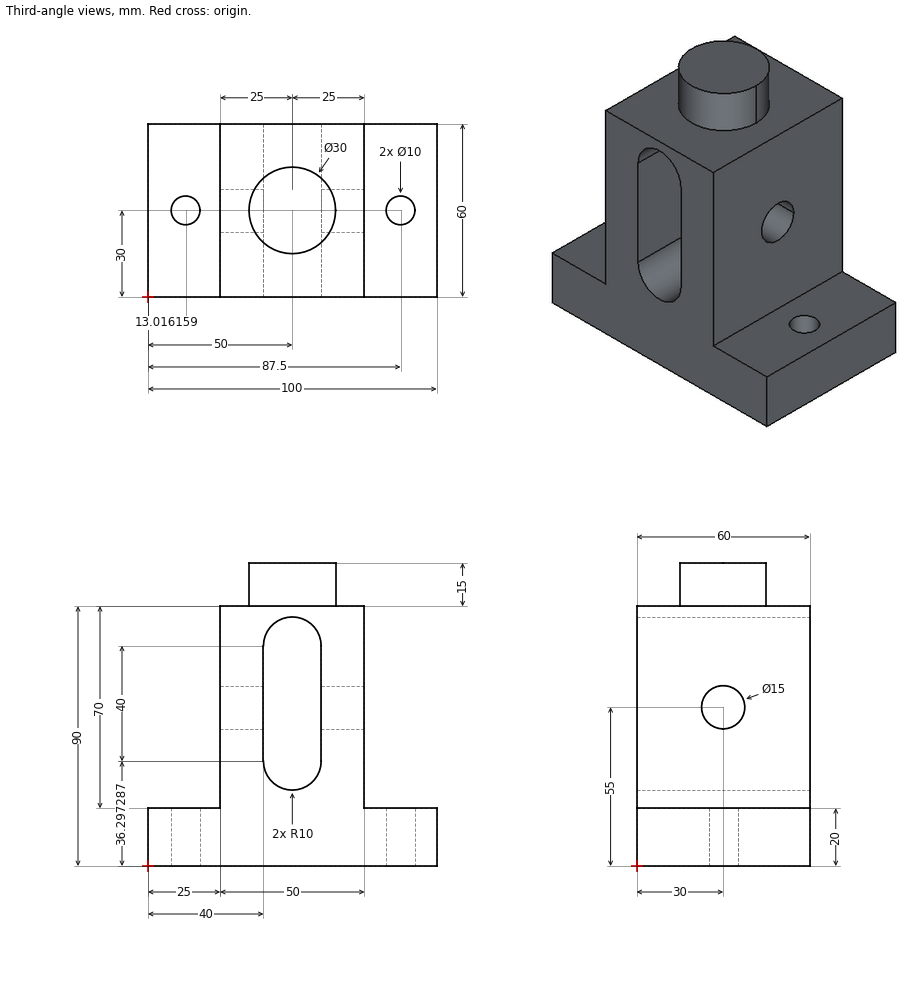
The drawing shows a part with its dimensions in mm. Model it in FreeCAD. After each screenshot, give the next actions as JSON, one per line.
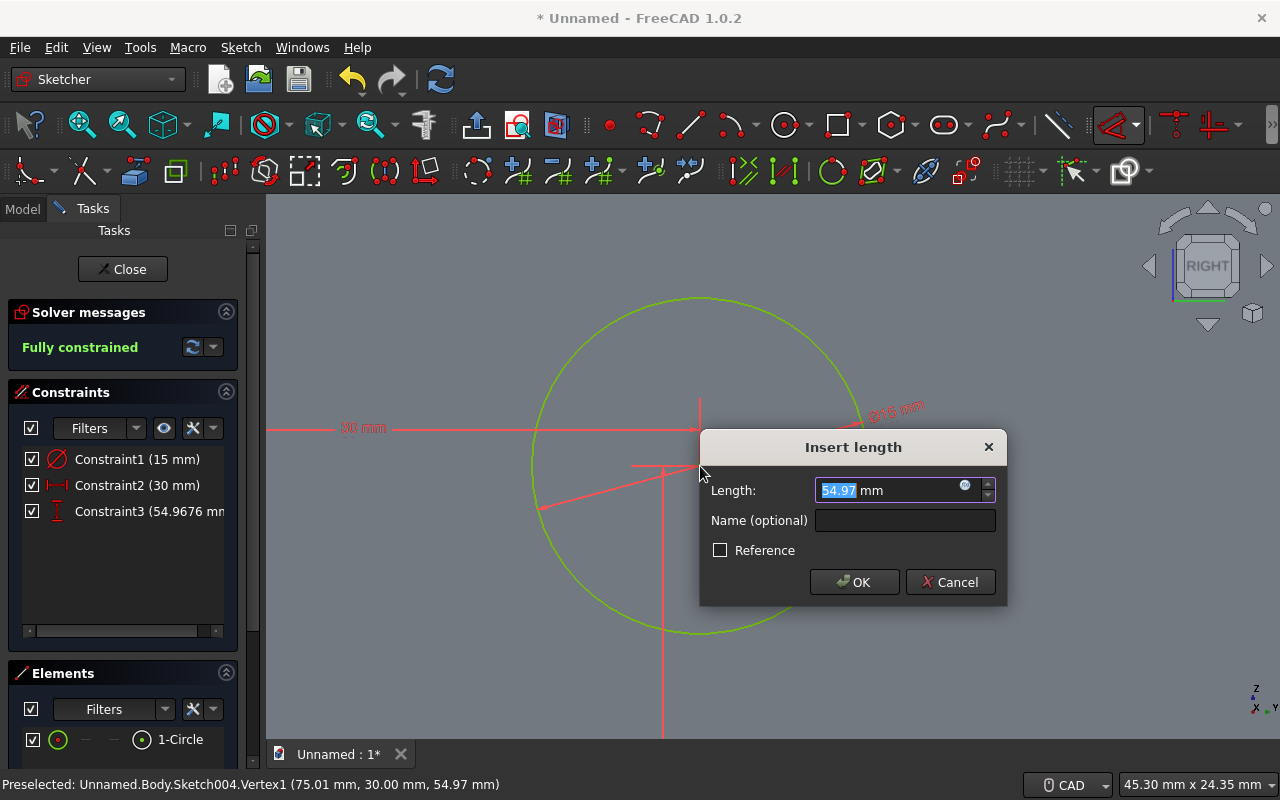
{"action": "type", "text": "55"}
{"action": "key", "text": "Return"}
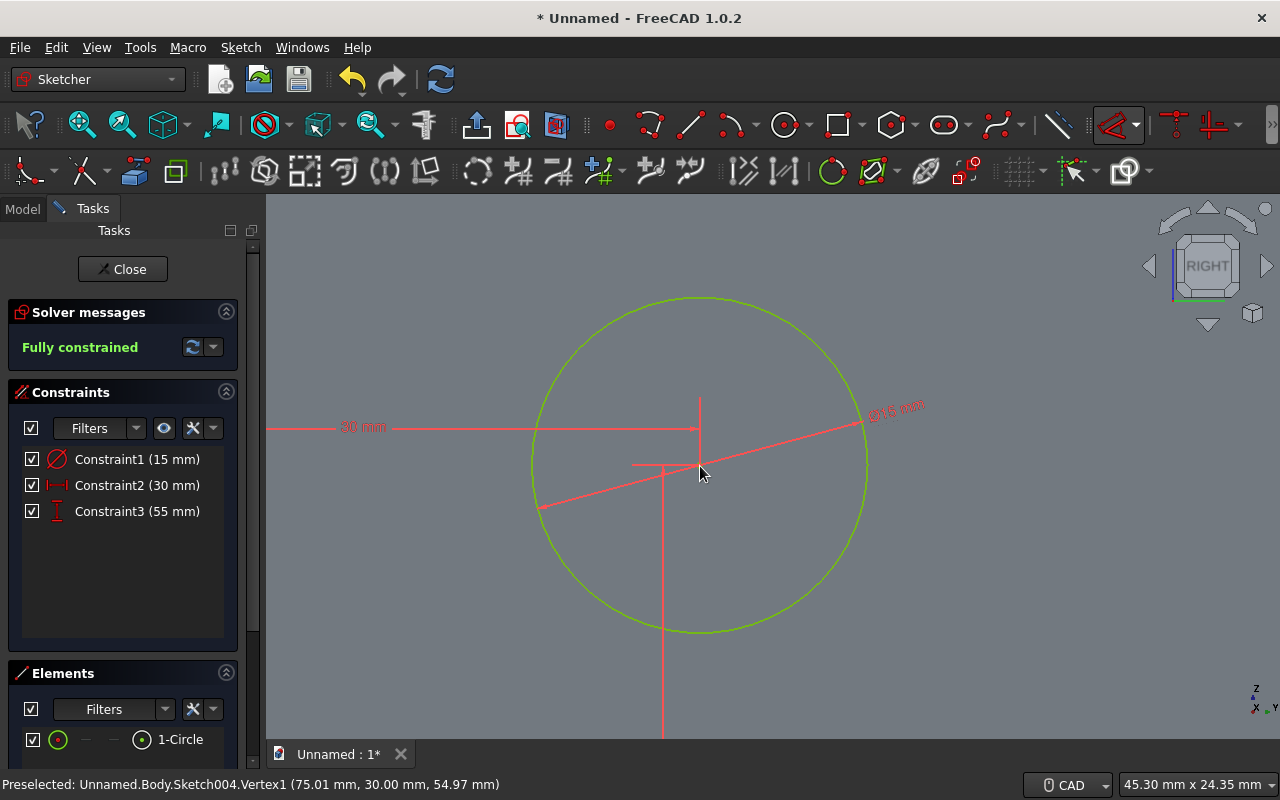
{"action": "left_click", "coordinate": [123, 269]}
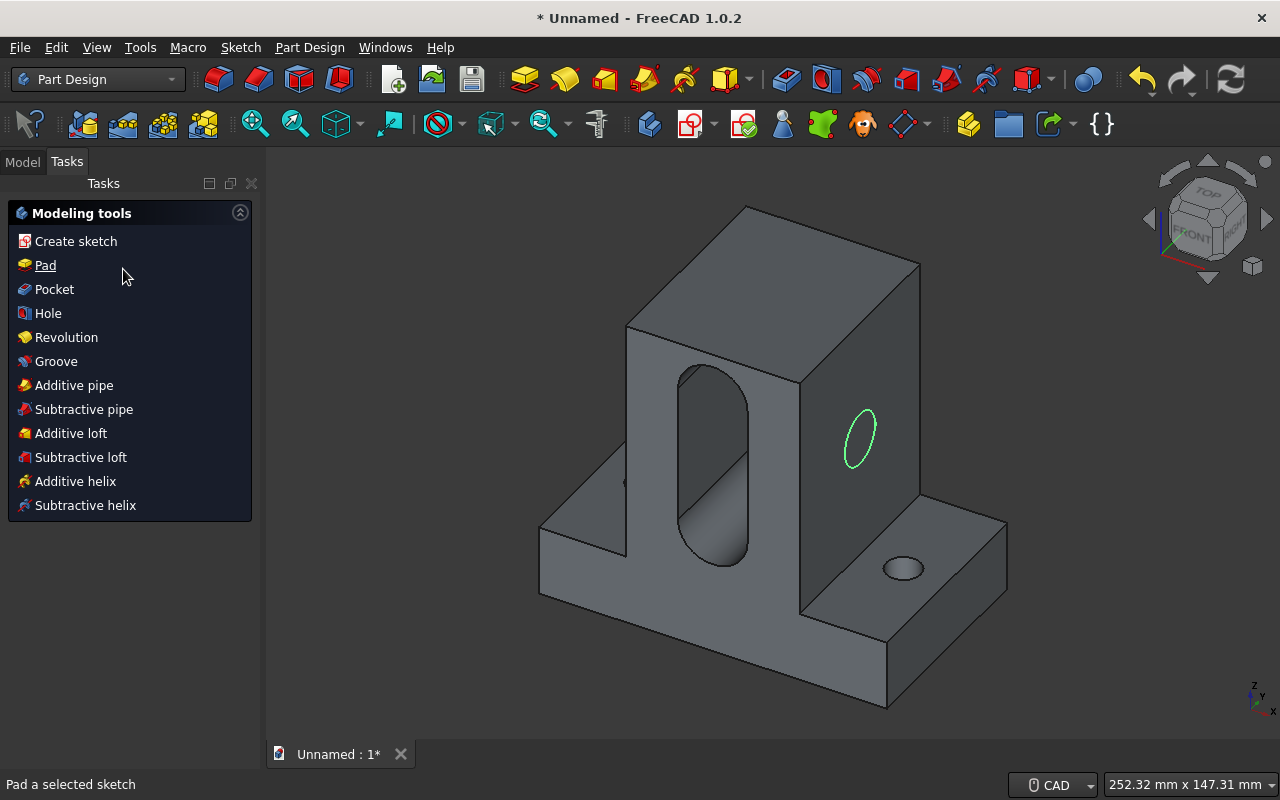
{"action": "left_click", "coordinate": [788, 80]}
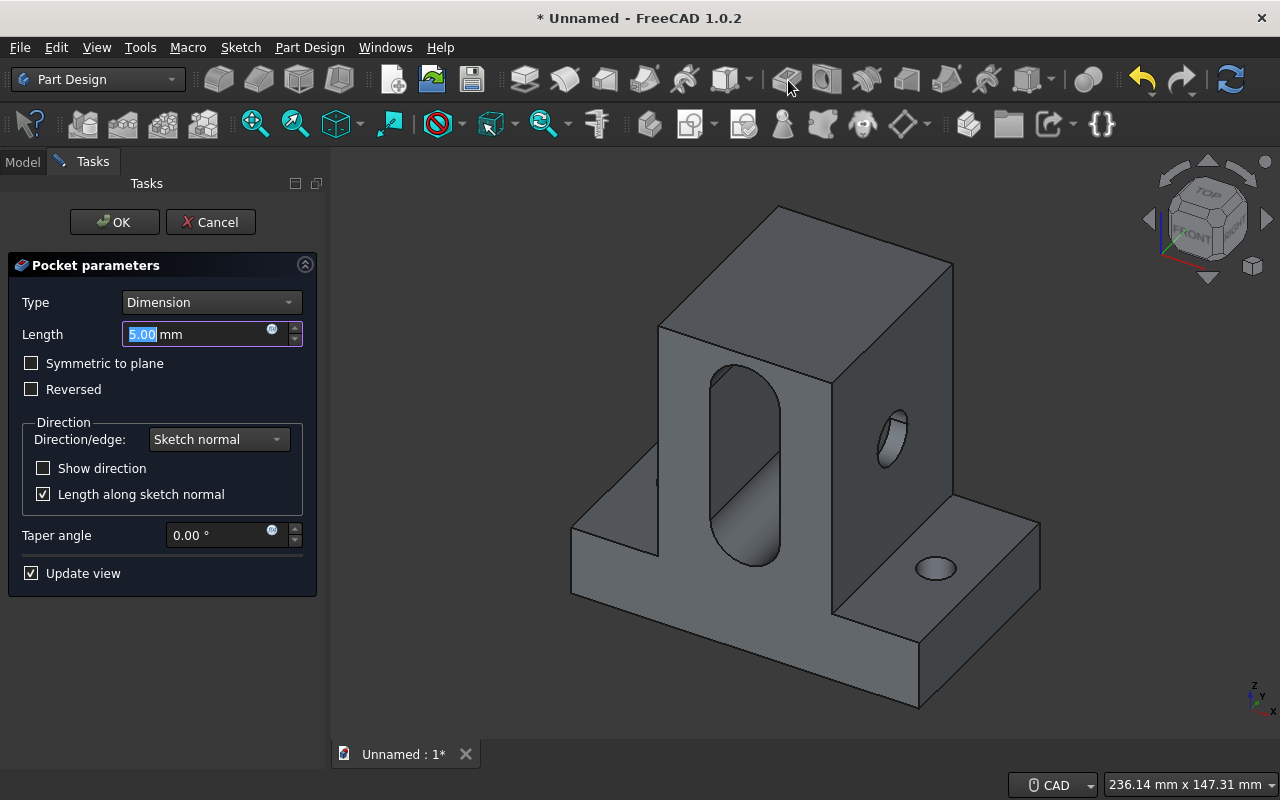
{"action": "type", "text": "25"}
{"action": "key", "text": "Tab"}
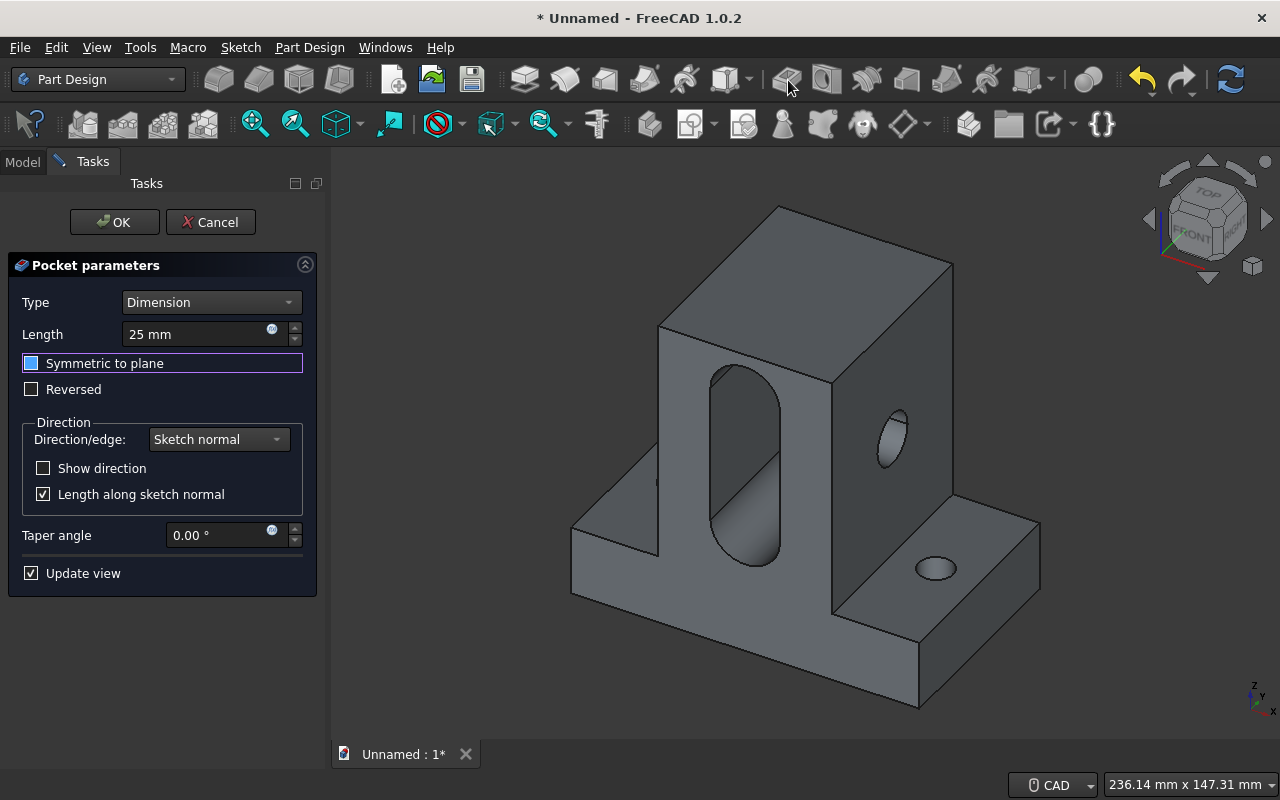
{"action": "left_click", "coordinate": [115, 222]}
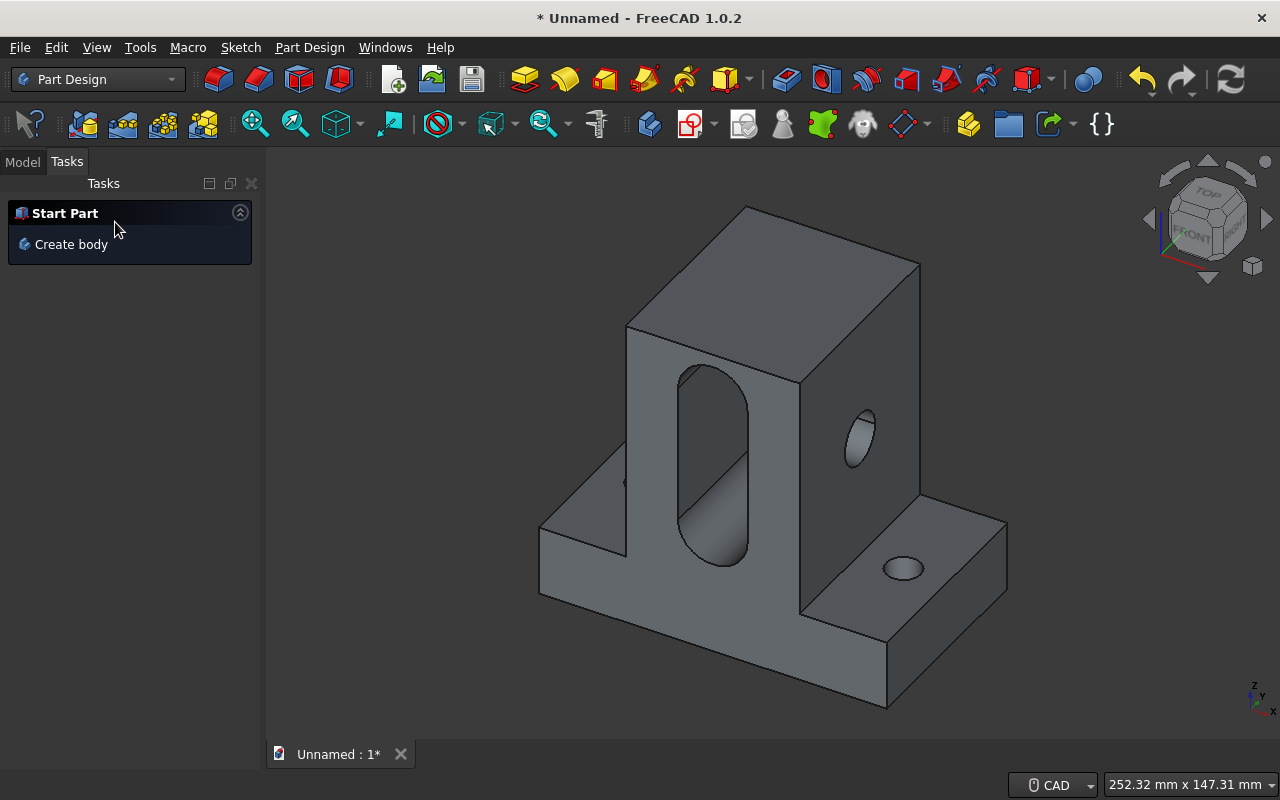
{"action": "left_click", "coordinate": [23, 161]}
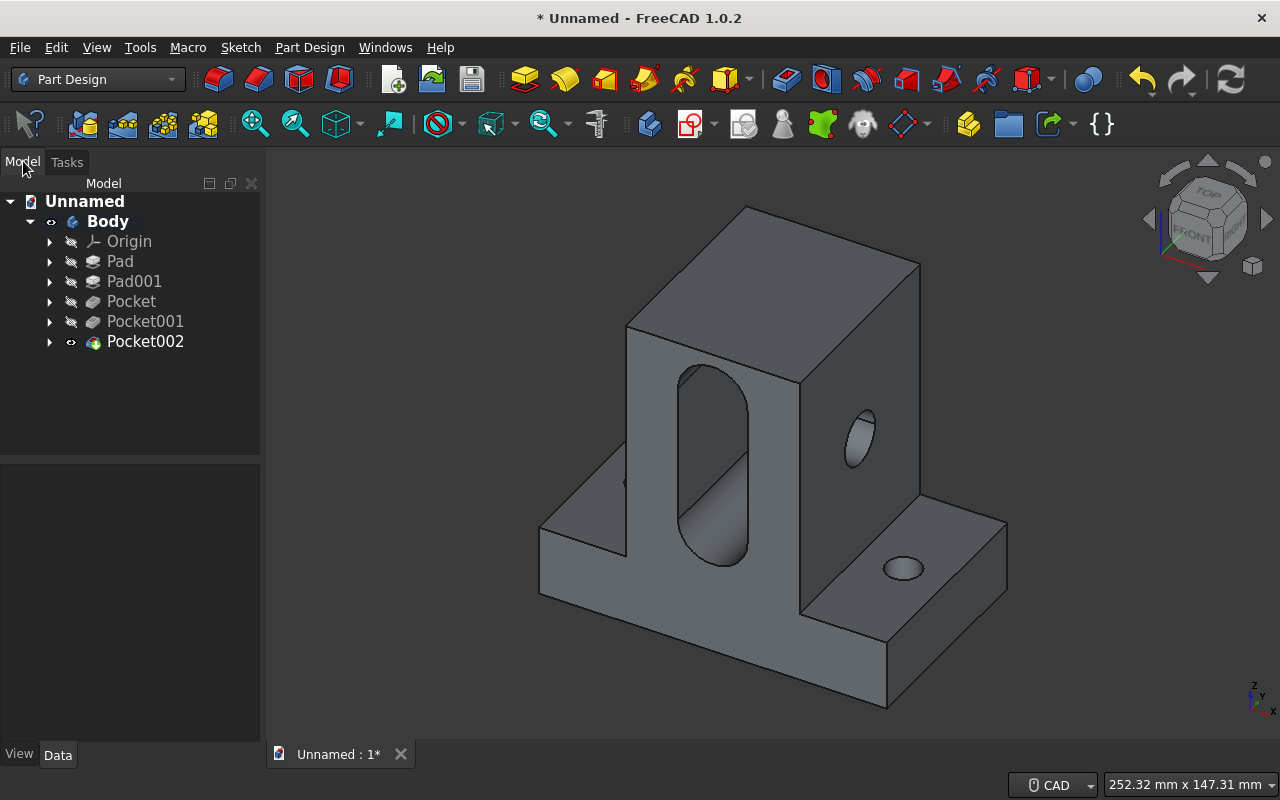
{"action": "left_click", "coordinate": [50, 242]}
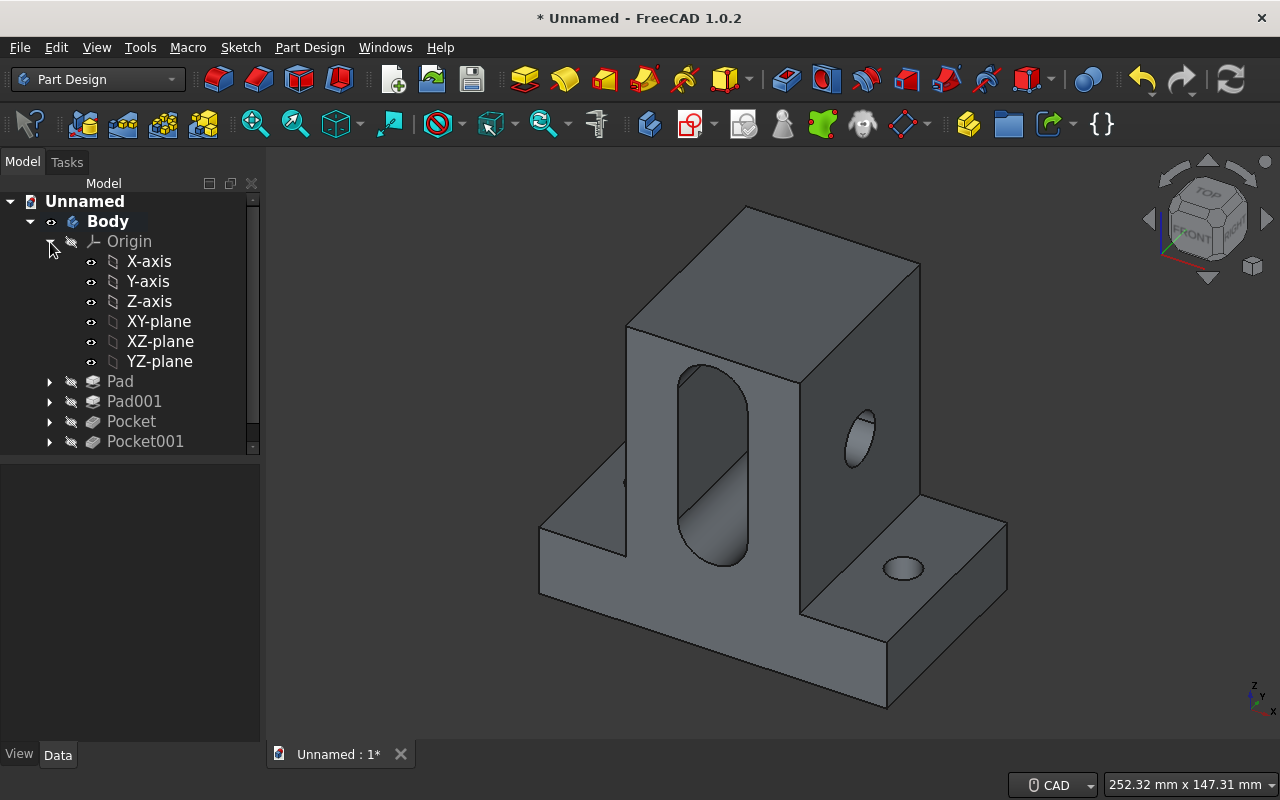
{"action": "left_click", "coordinate": [136, 362]}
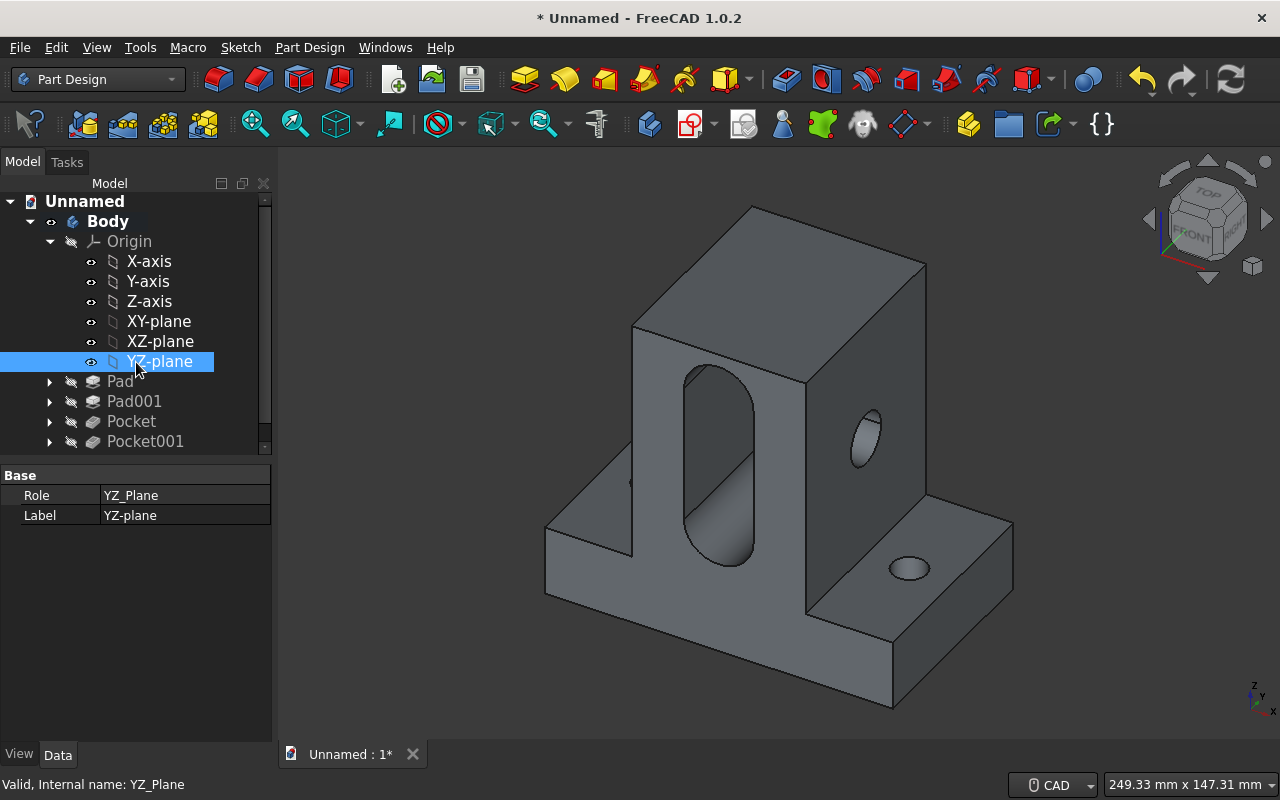
{"action": "left_click", "coordinate": [904, 124]}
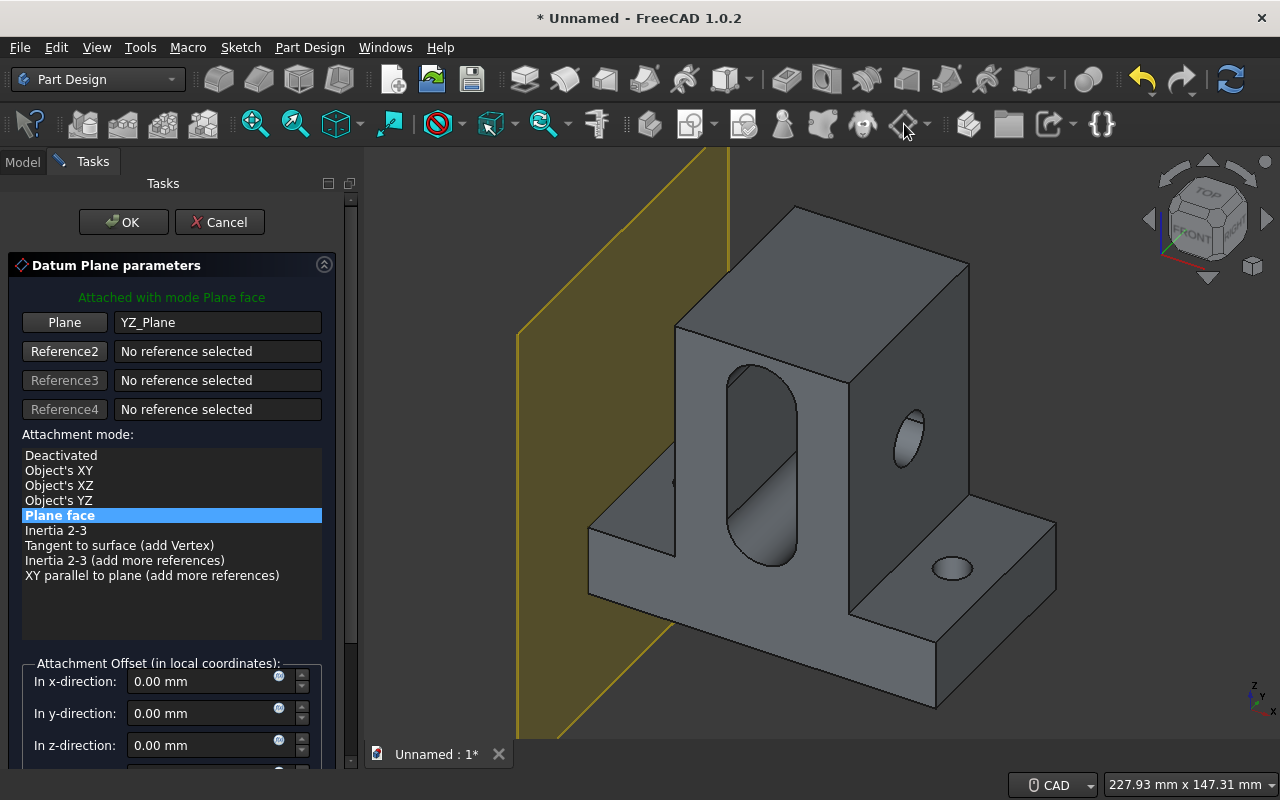
{"action": "triple_click", "coordinate": [210, 745]}